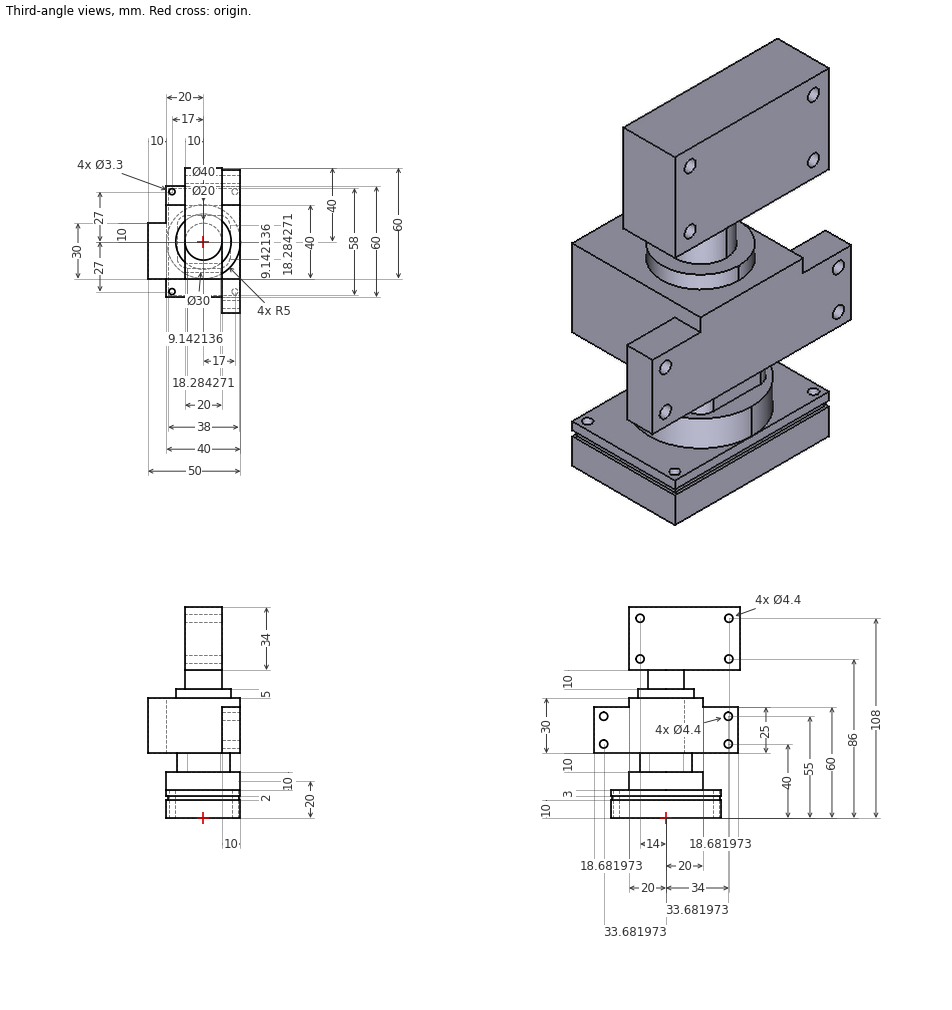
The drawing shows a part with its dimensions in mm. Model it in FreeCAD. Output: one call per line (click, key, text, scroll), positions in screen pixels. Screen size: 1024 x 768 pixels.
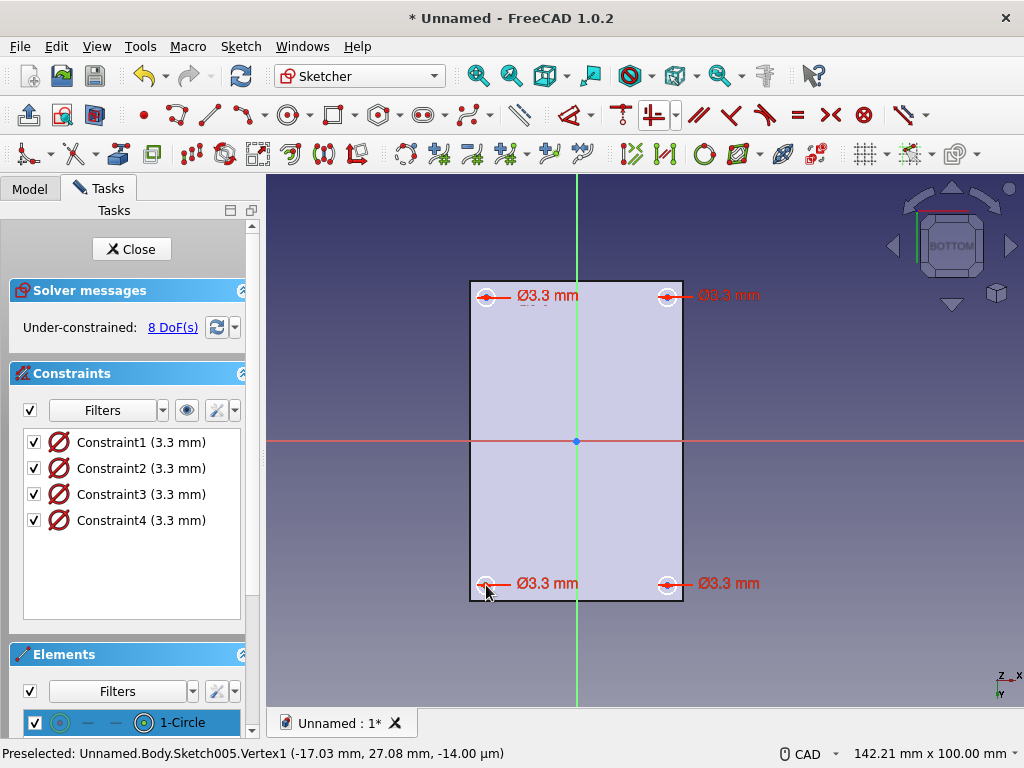
click(486, 298)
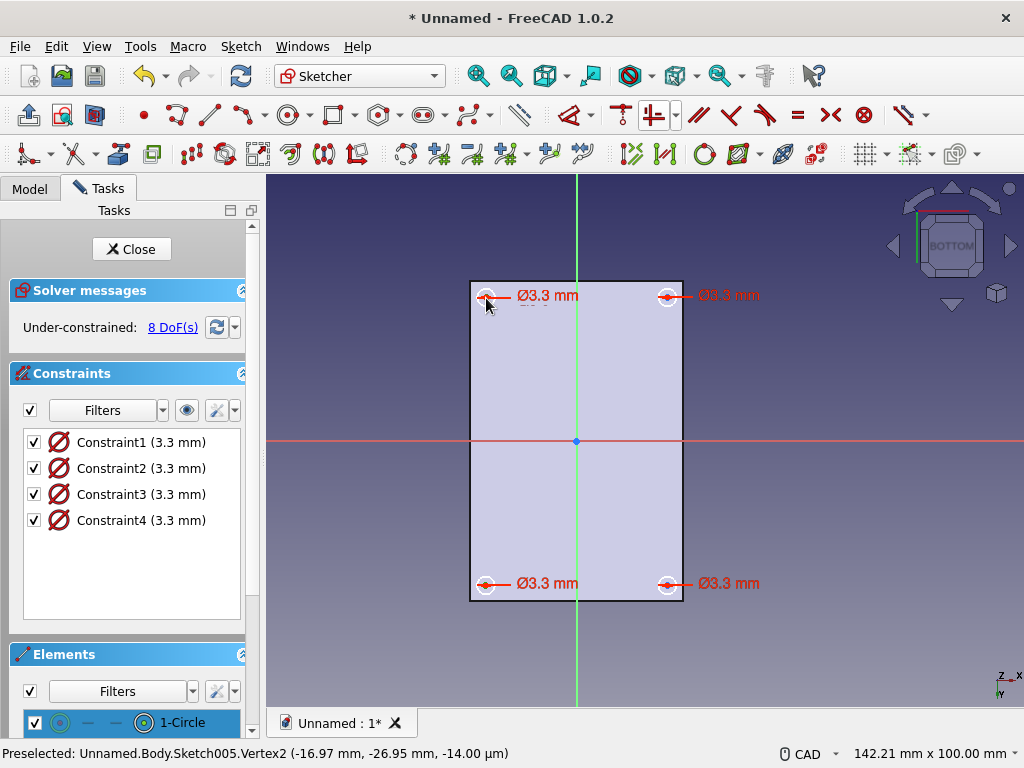
key(v)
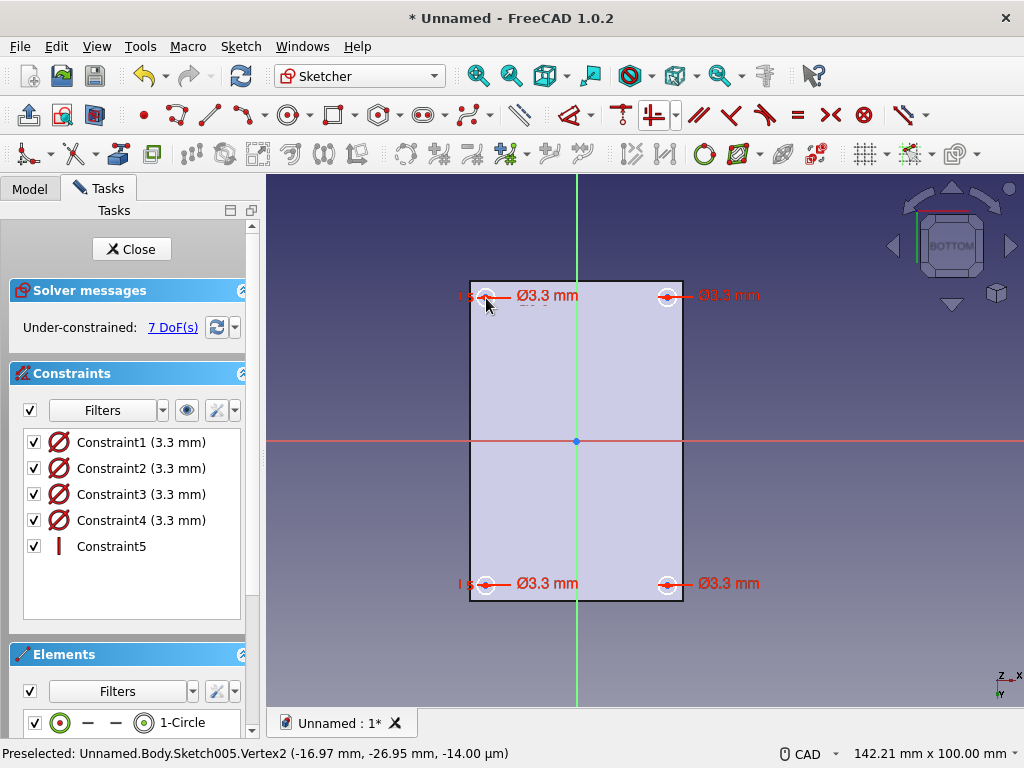
click(486, 298)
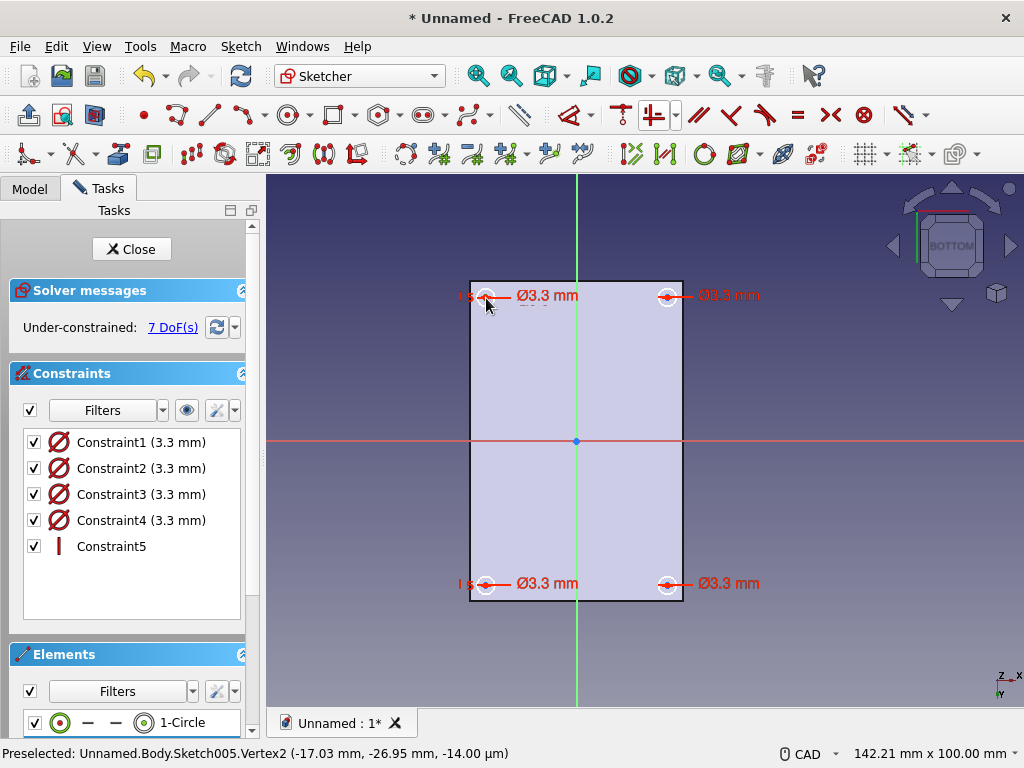
click(667, 297)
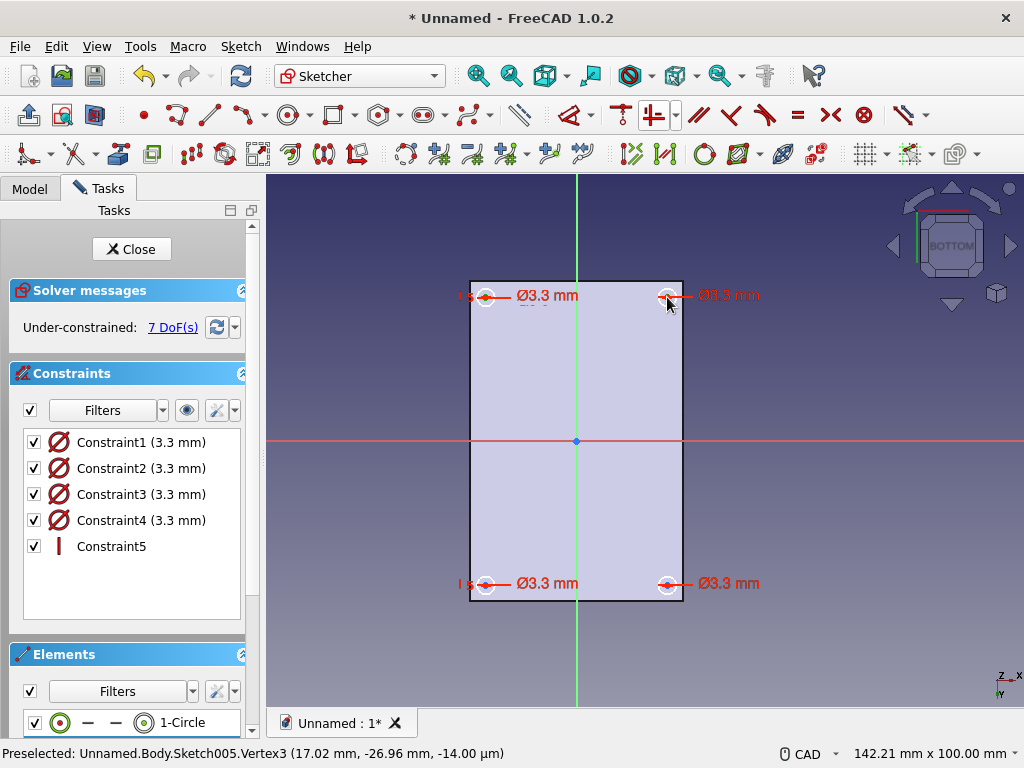
key(h)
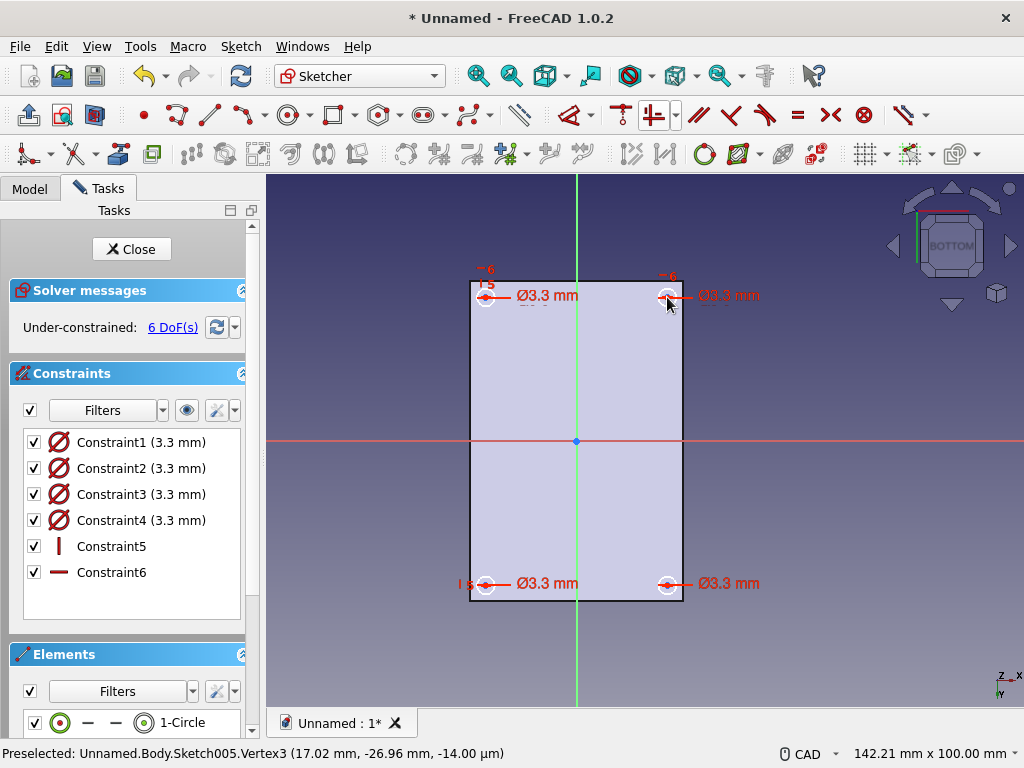
click(667, 298)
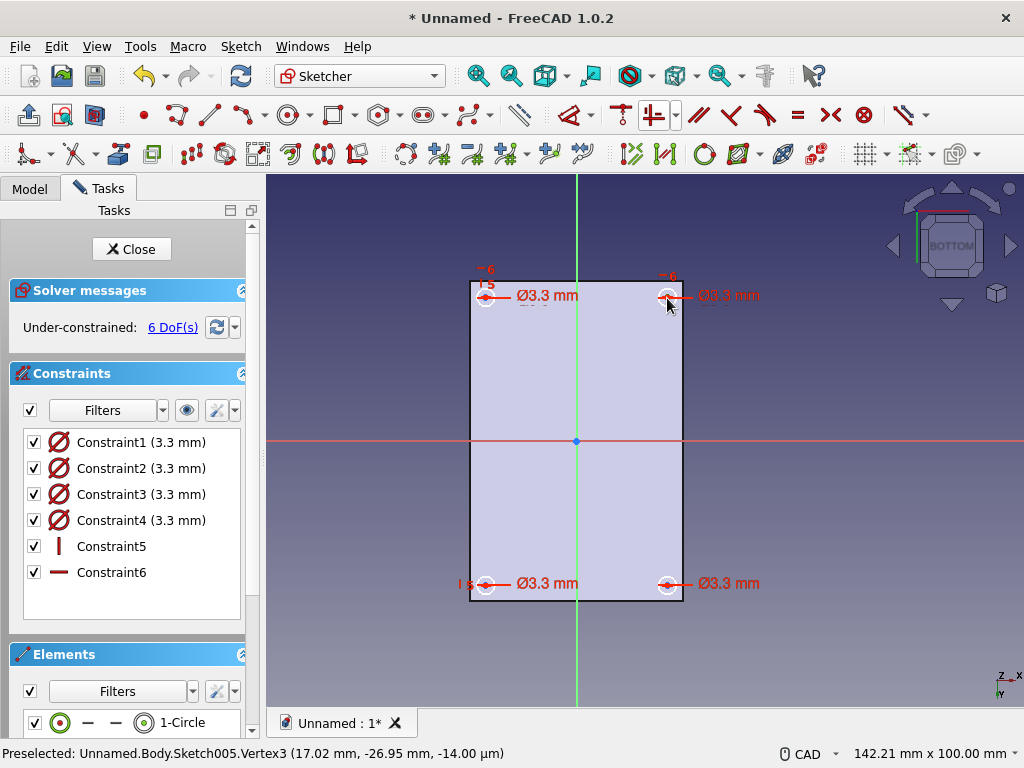
click(667, 585)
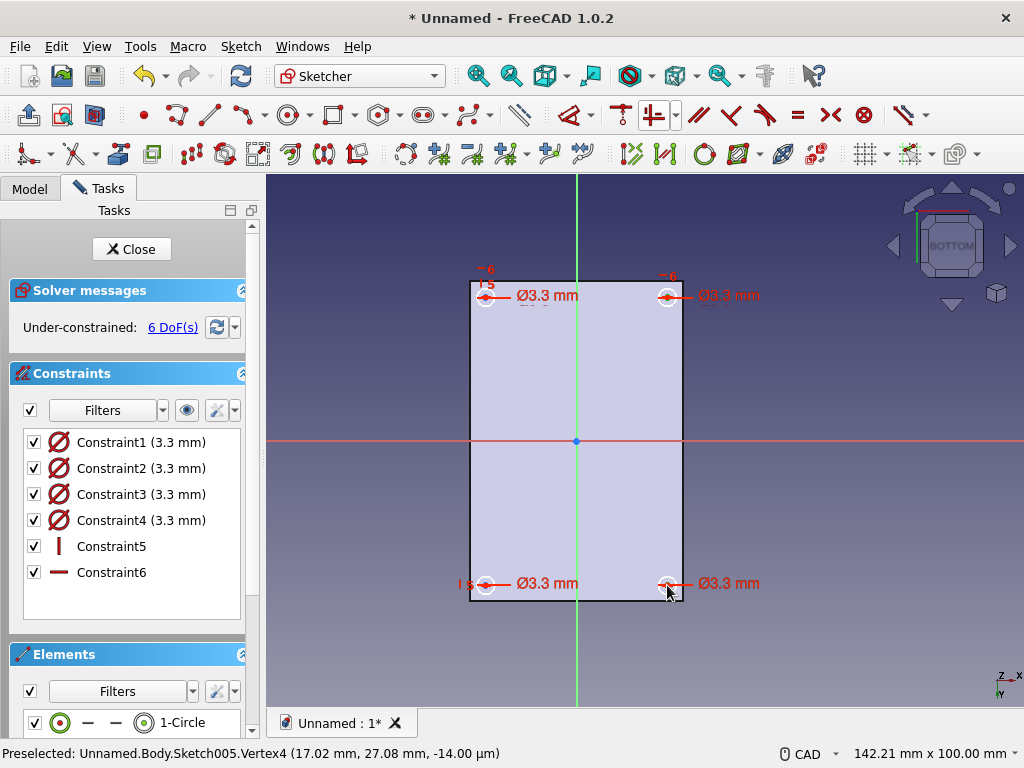
key(v)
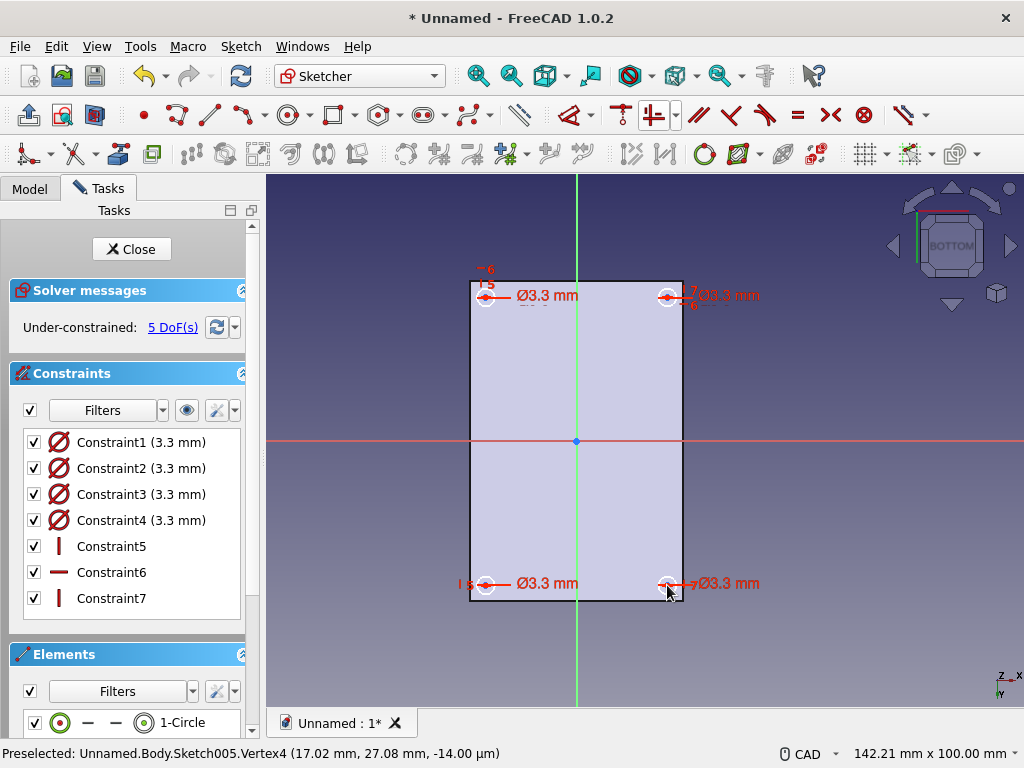
click(486, 585)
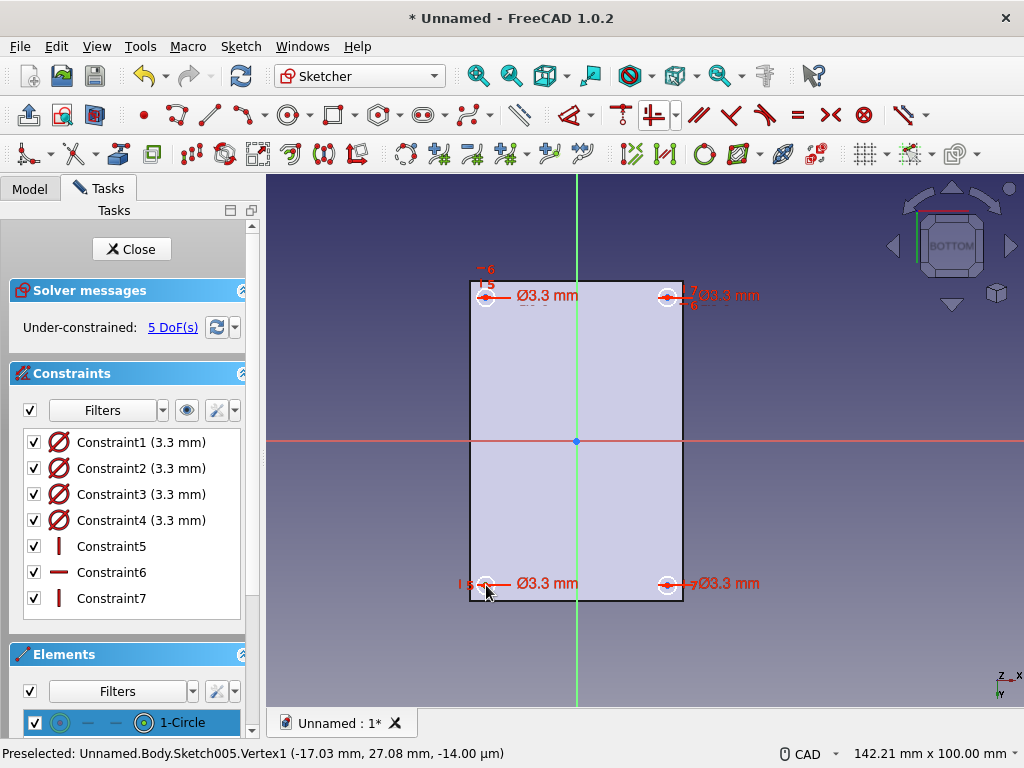
click(667, 585)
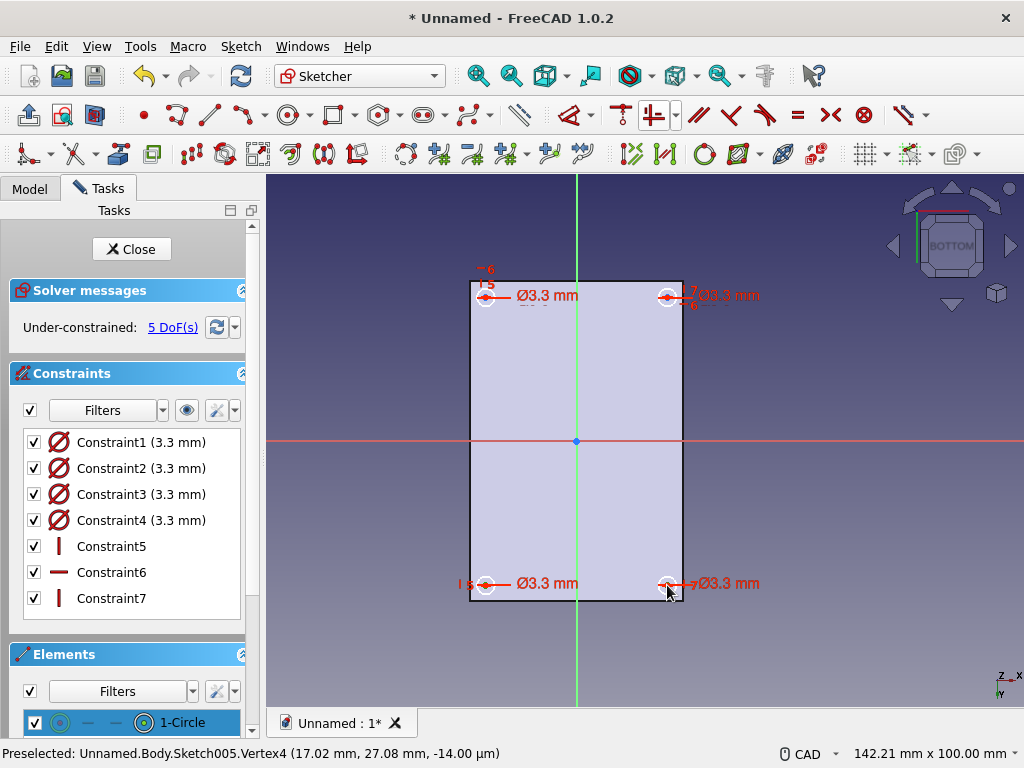
key(h)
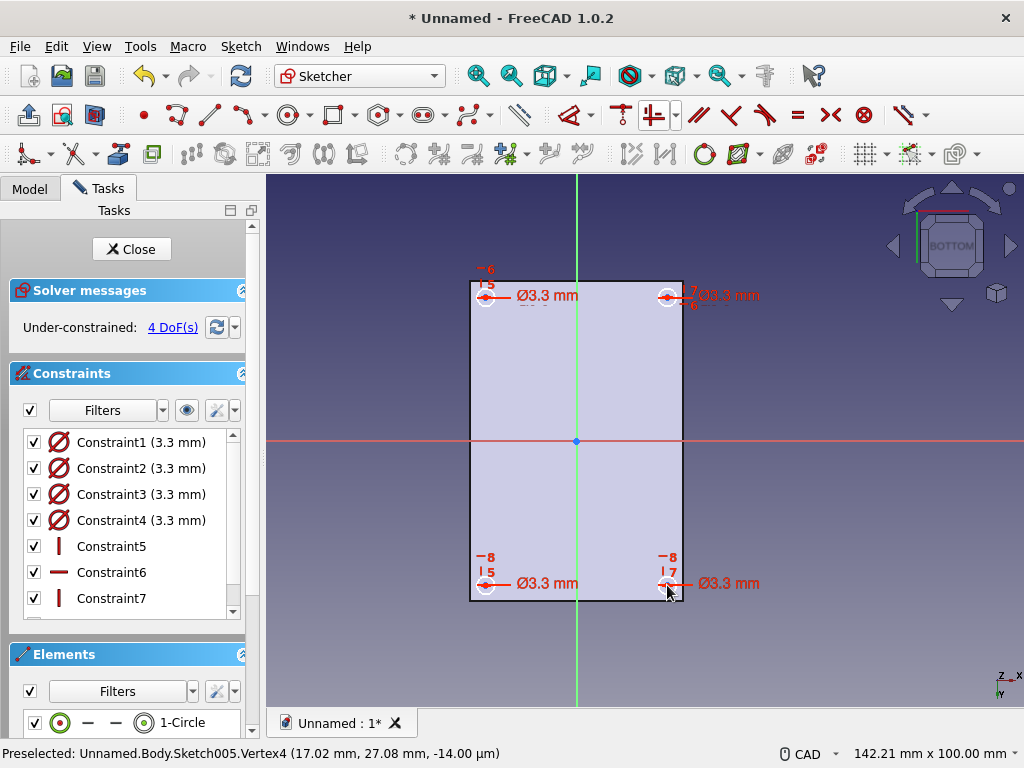
key(d)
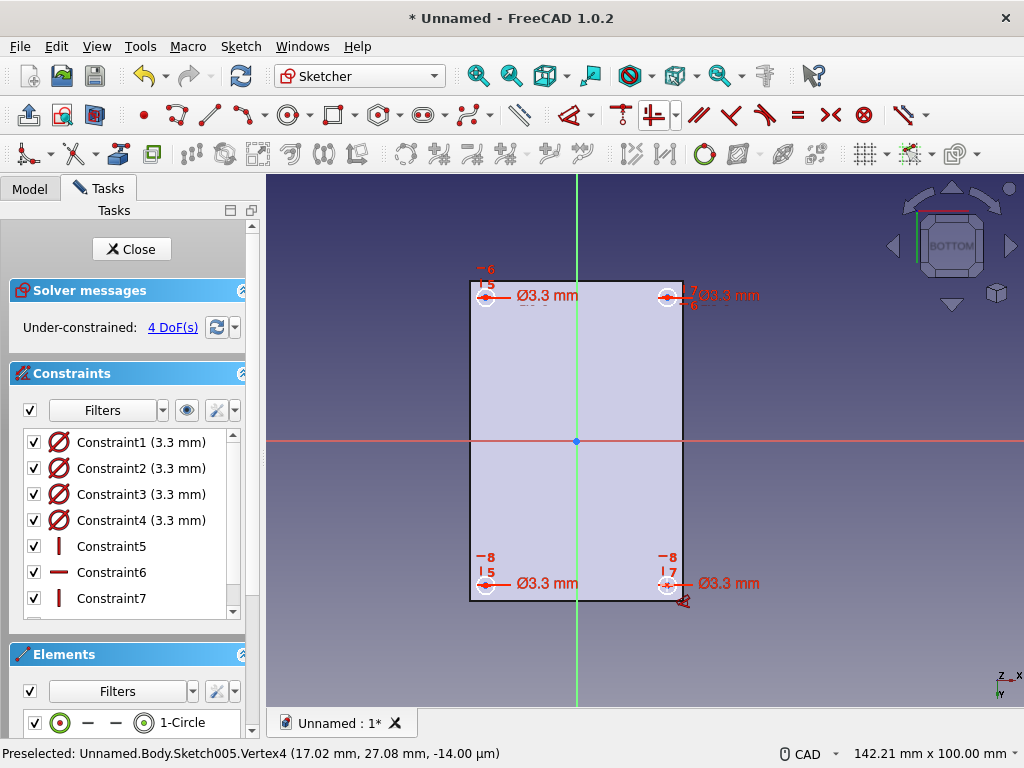
click(486, 585)
click(531, 619)